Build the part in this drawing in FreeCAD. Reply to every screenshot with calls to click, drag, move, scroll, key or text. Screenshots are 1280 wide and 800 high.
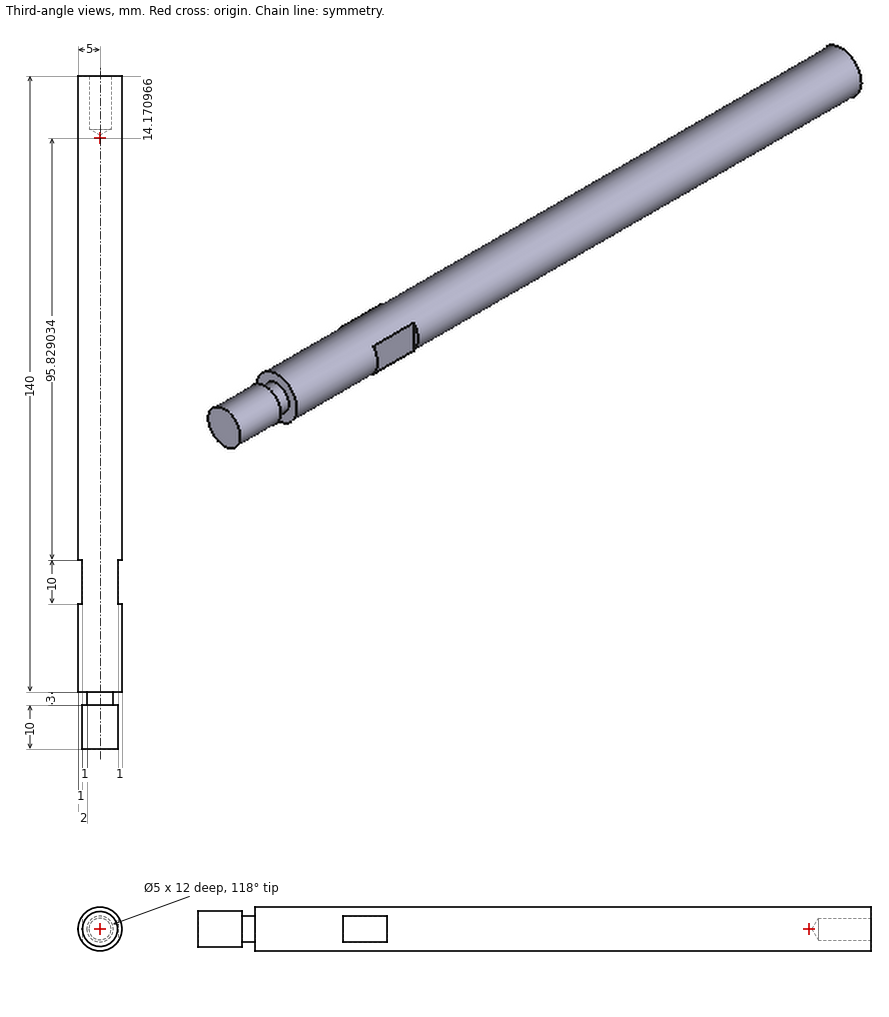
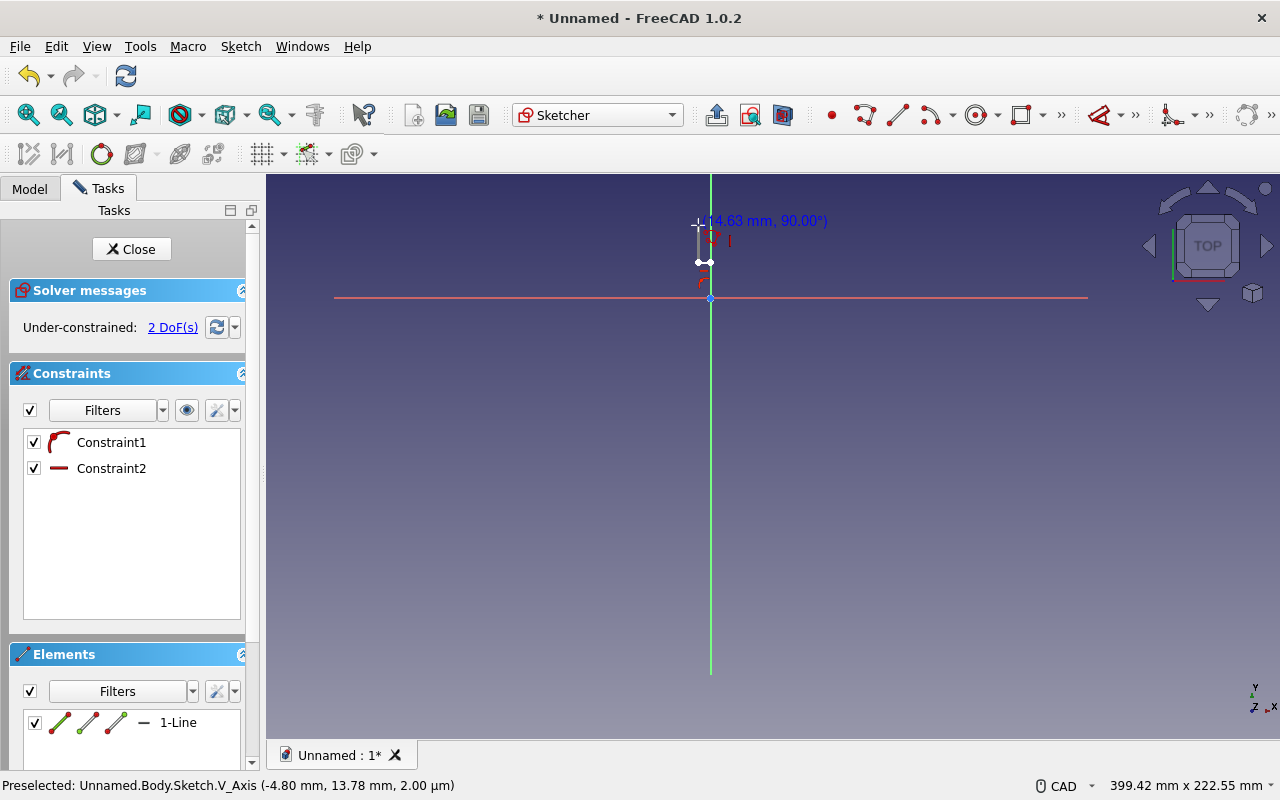
scroll(698, 618, up, 2)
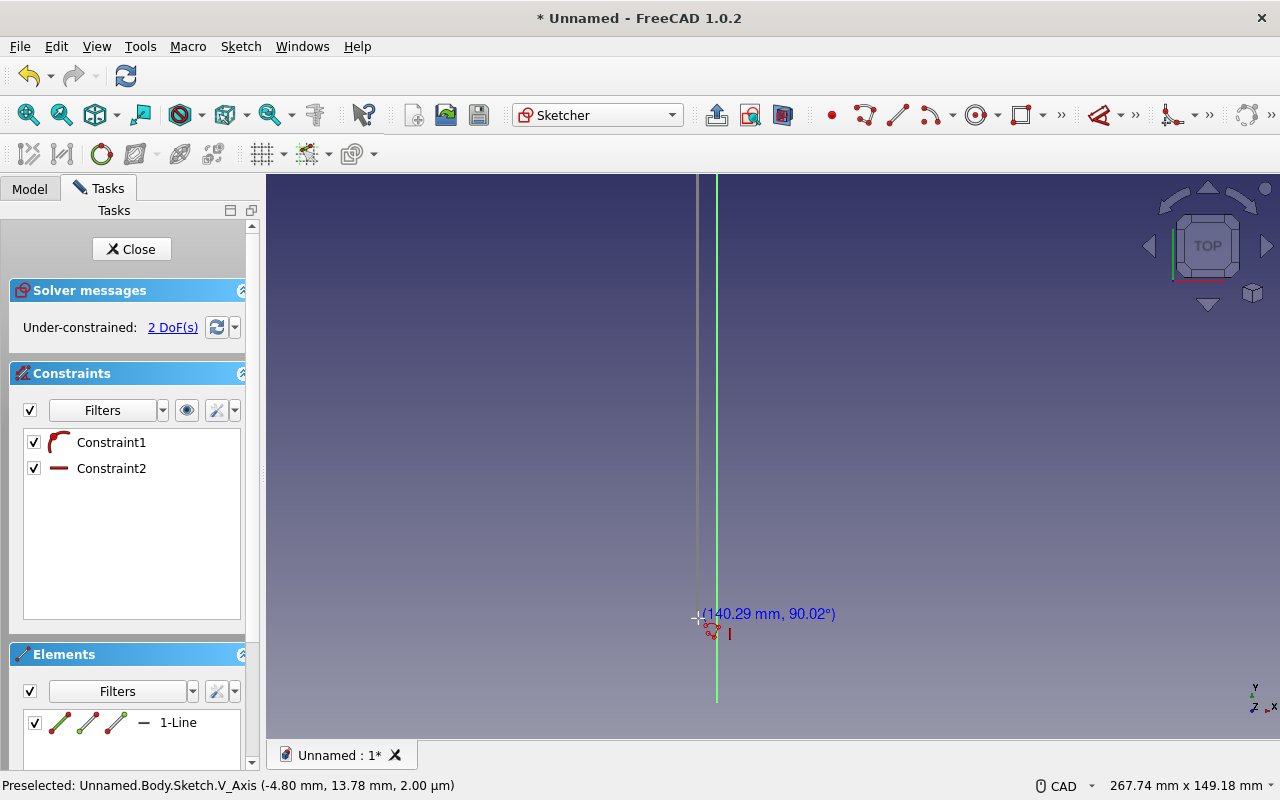
click(698, 617)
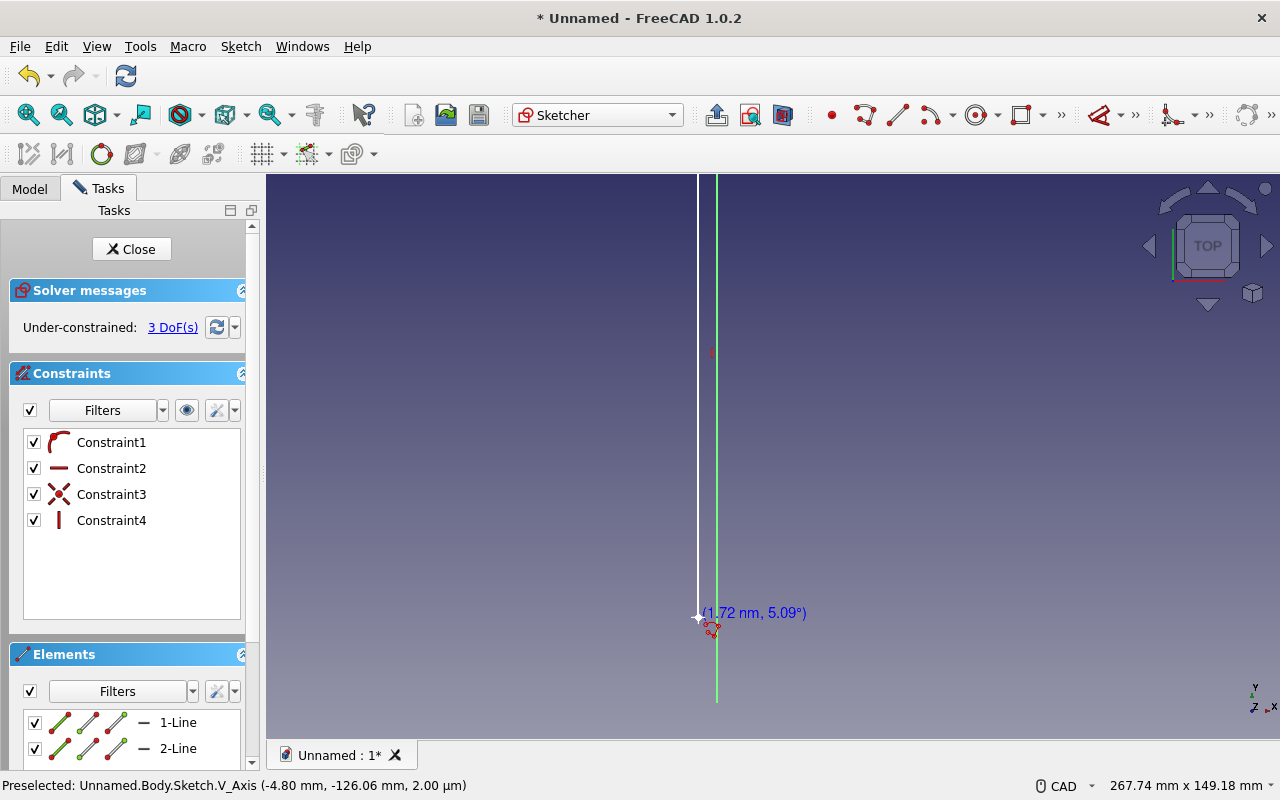
scroll(706, 617, up, 4)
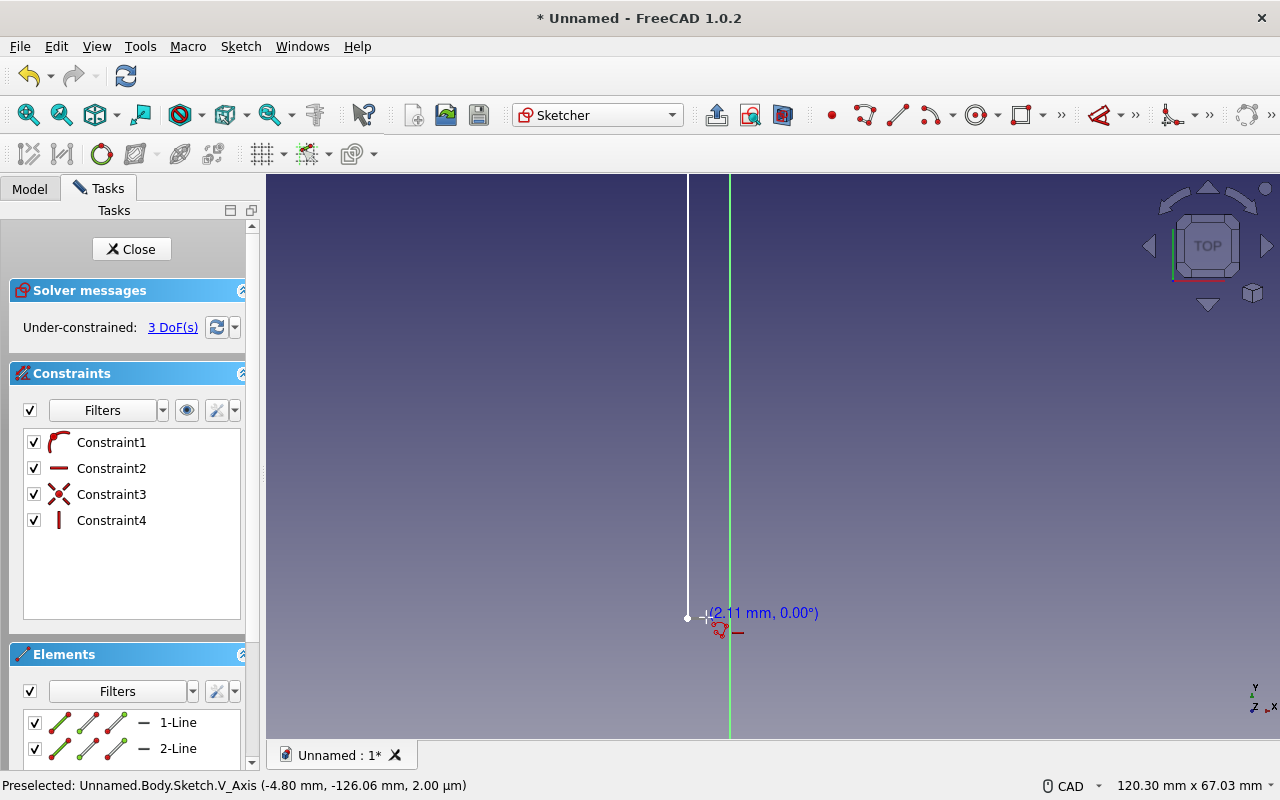
click(705, 616)
click(705, 642)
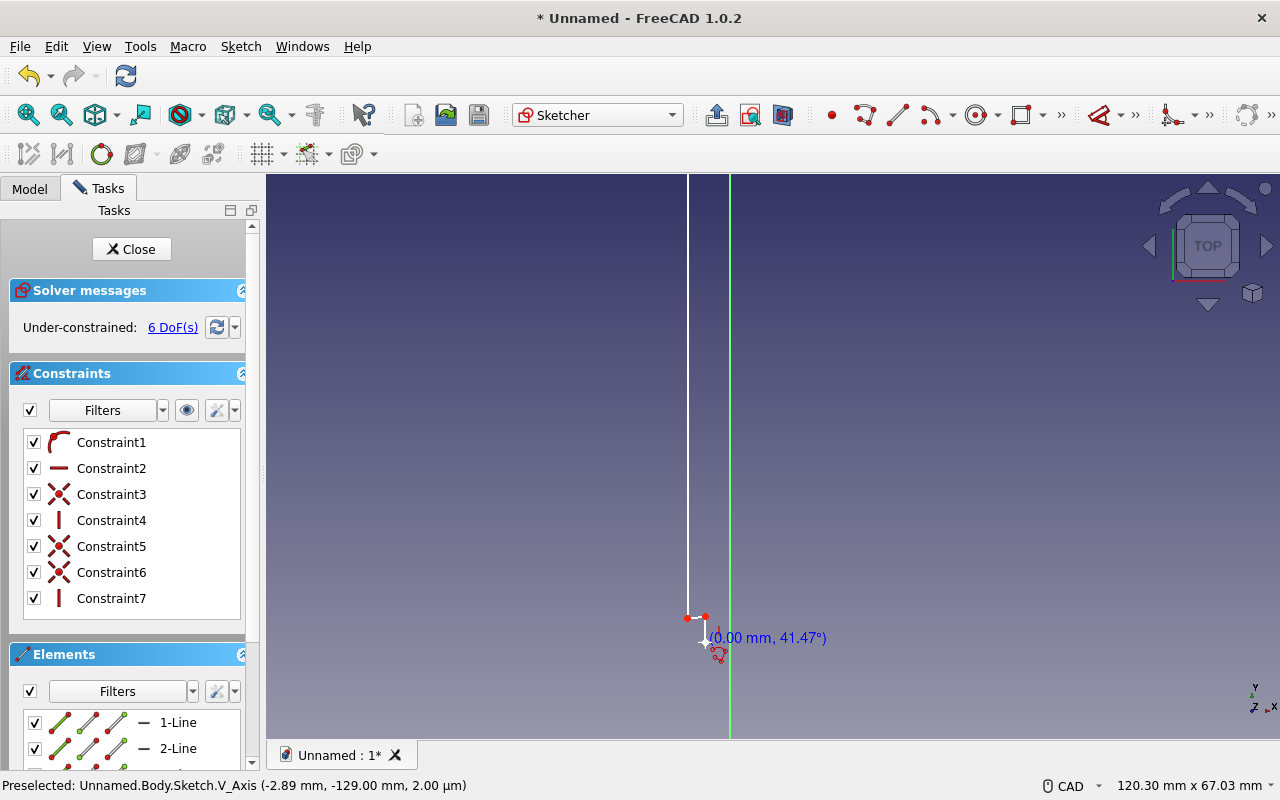
scroll(697, 642, up, 4)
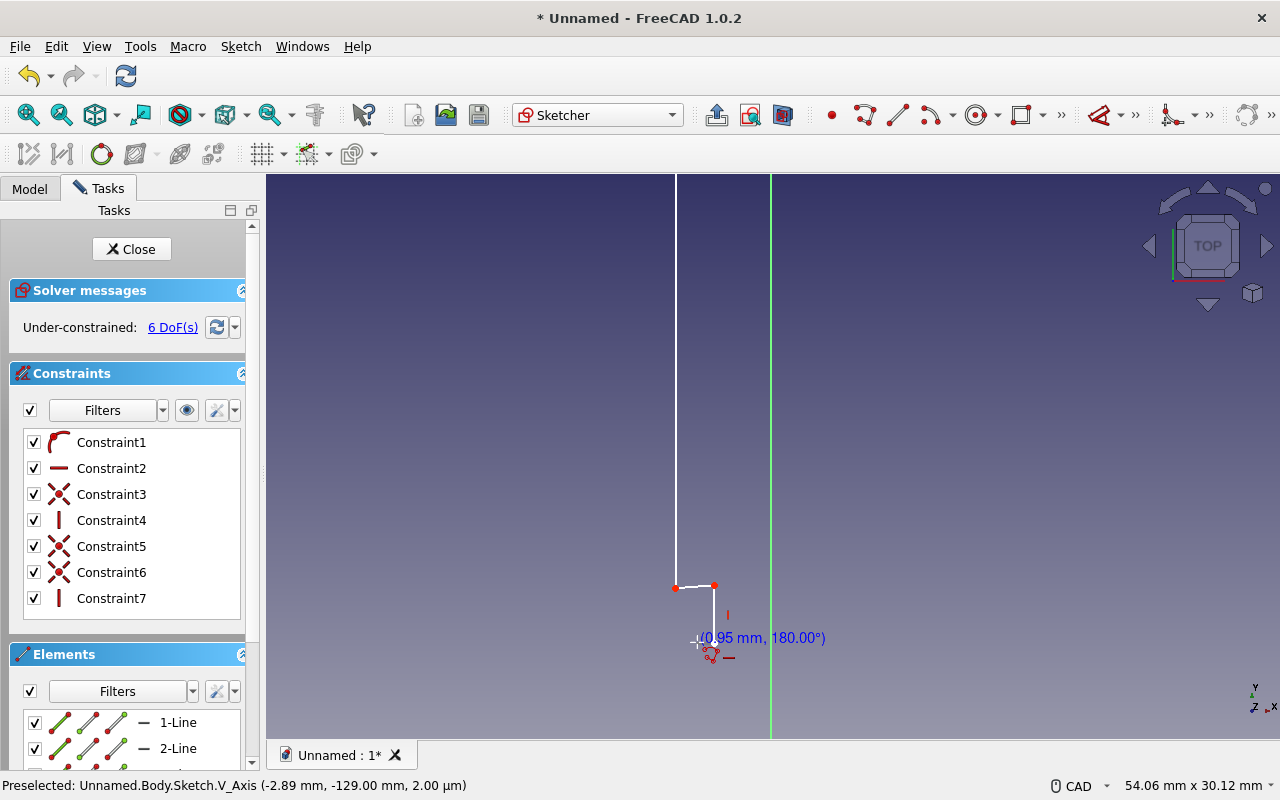
click(696, 641)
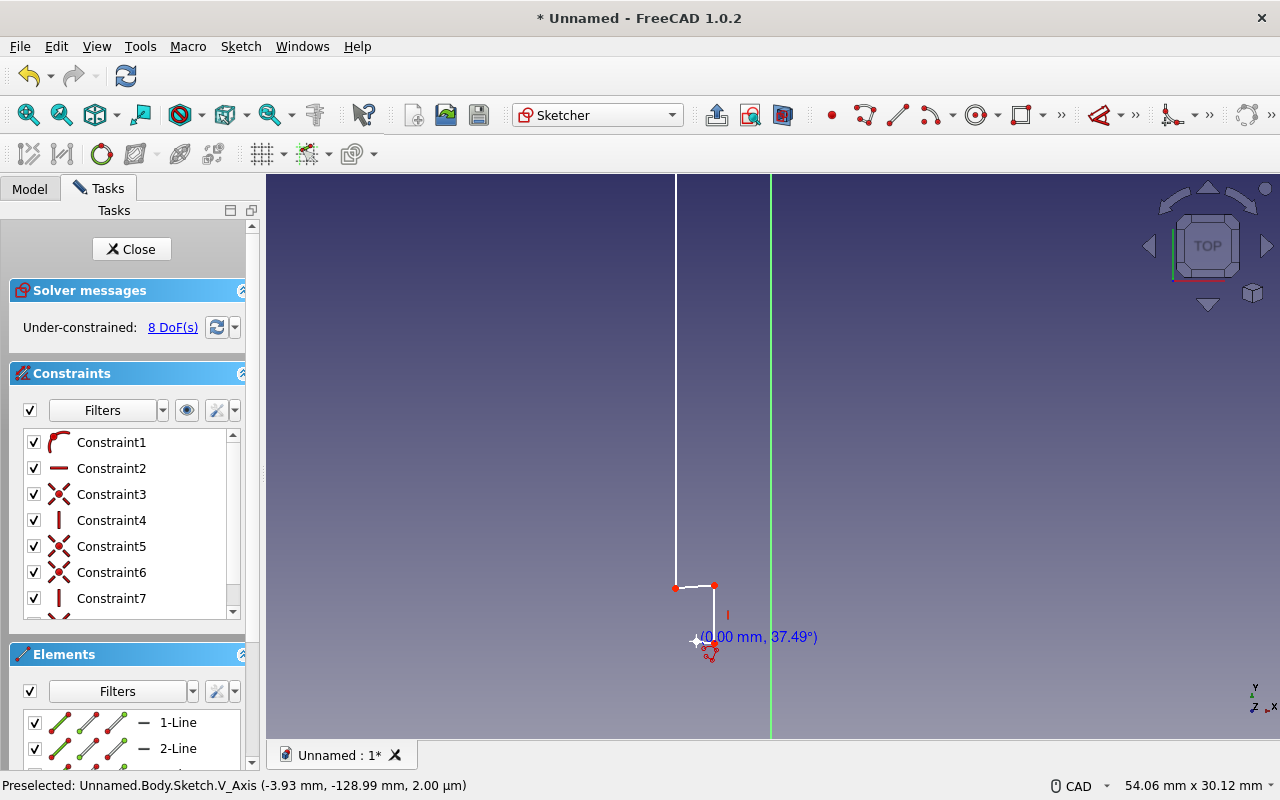
scroll(701, 623, down, 10)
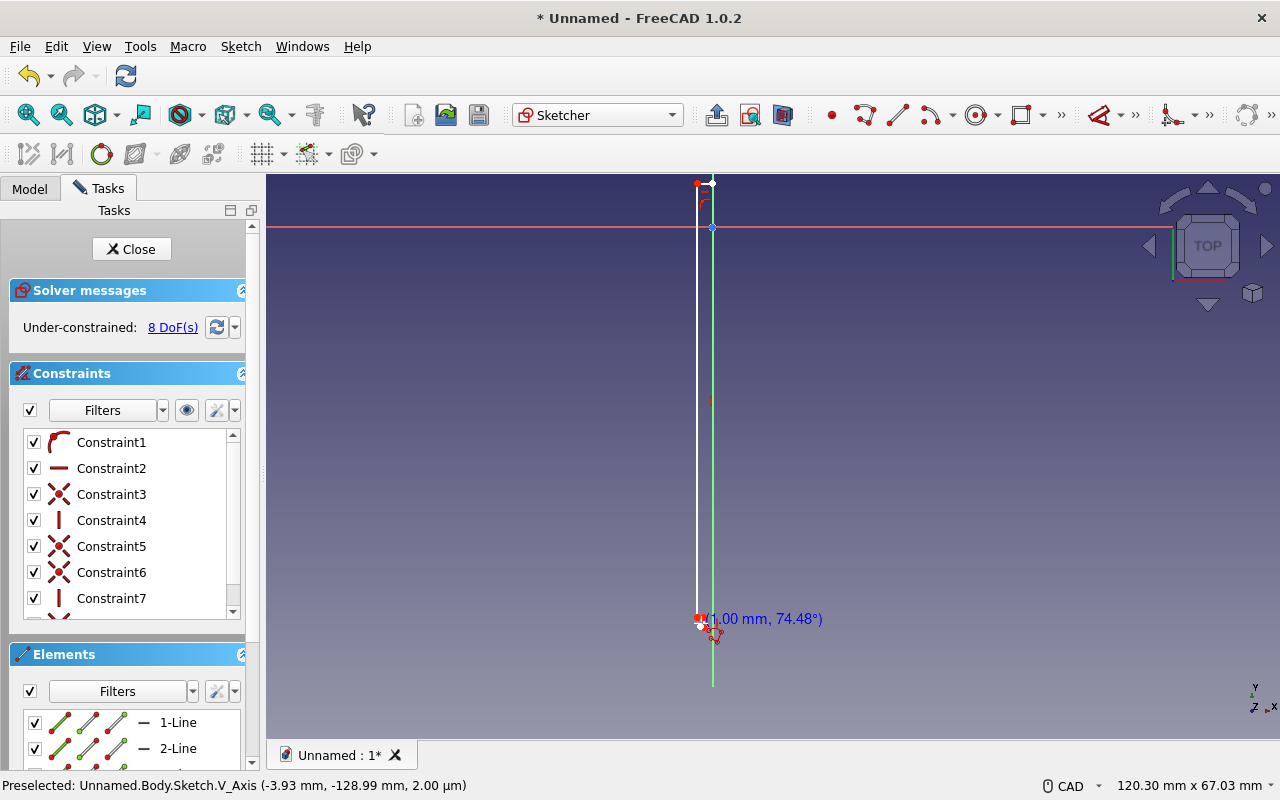
scroll(701, 651, up, 3)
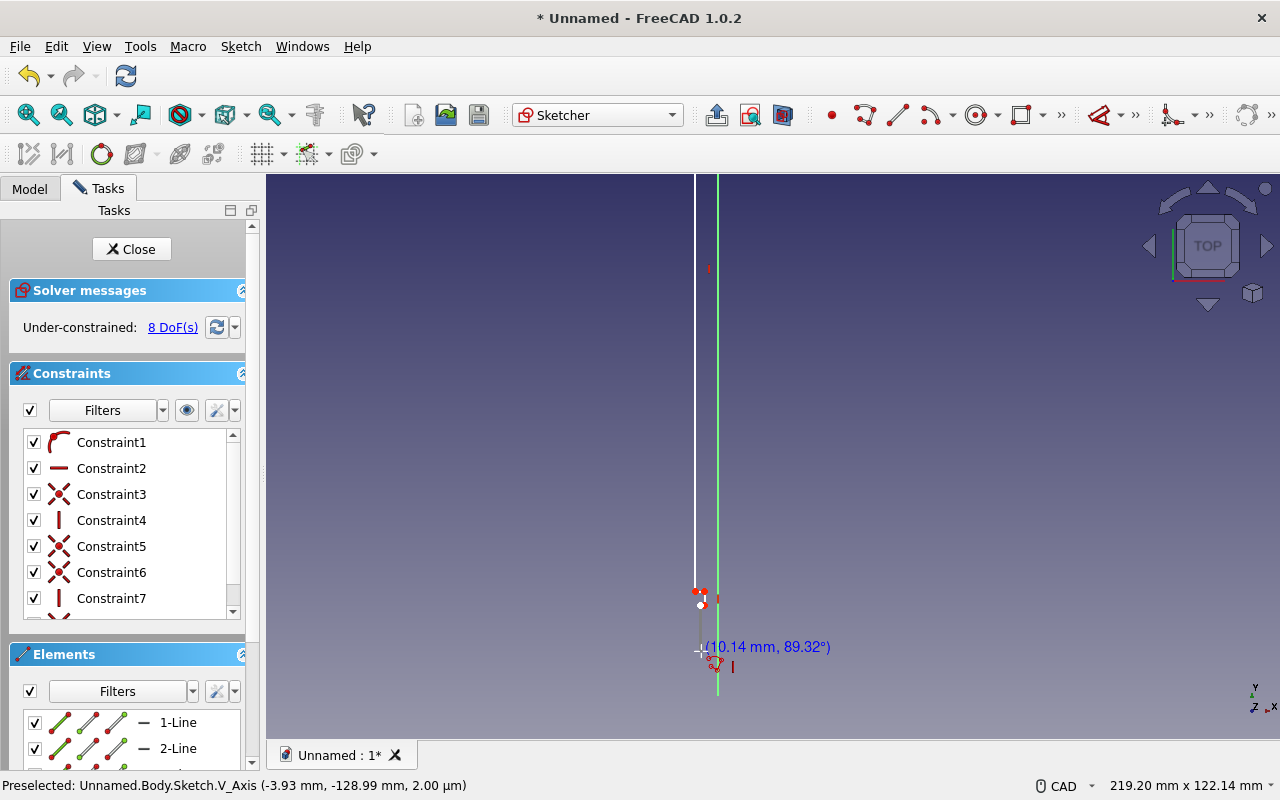
click(700, 651)
click(709, 651)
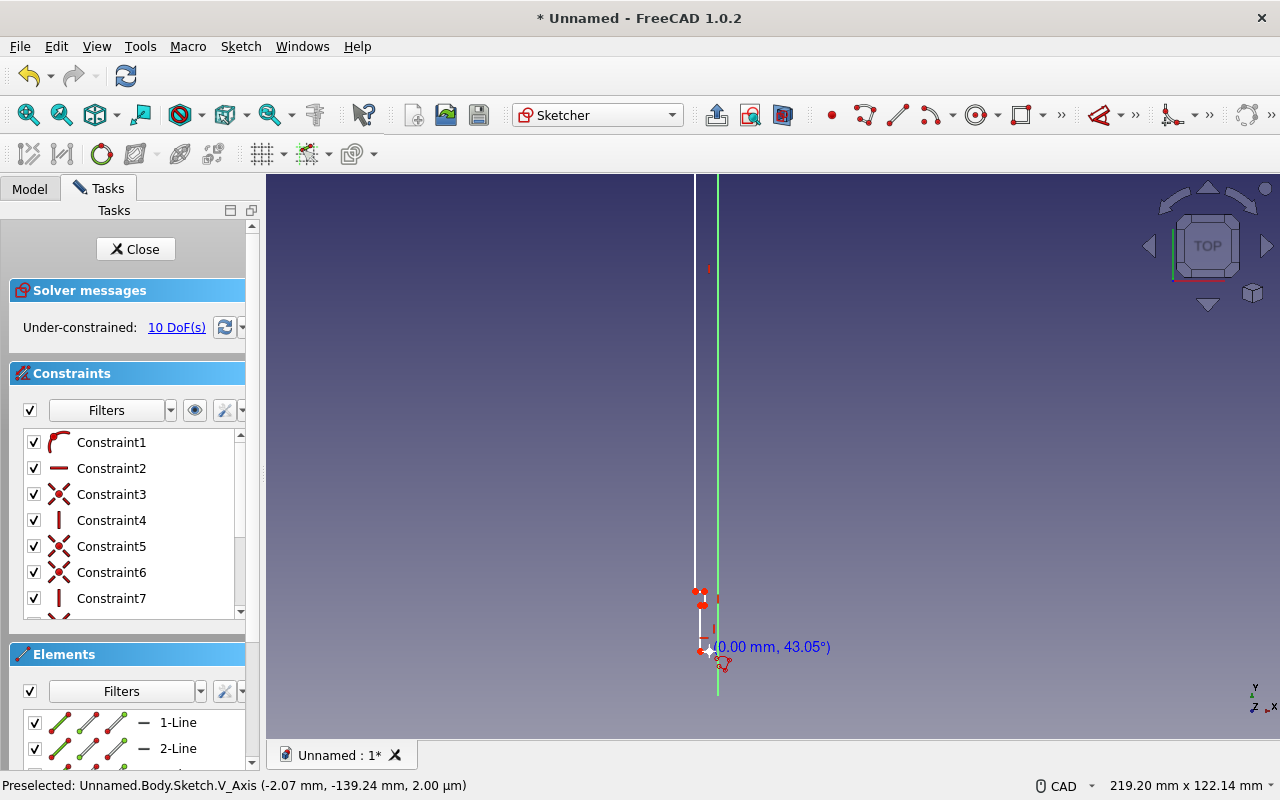
scroll(702, 650, down, 3)